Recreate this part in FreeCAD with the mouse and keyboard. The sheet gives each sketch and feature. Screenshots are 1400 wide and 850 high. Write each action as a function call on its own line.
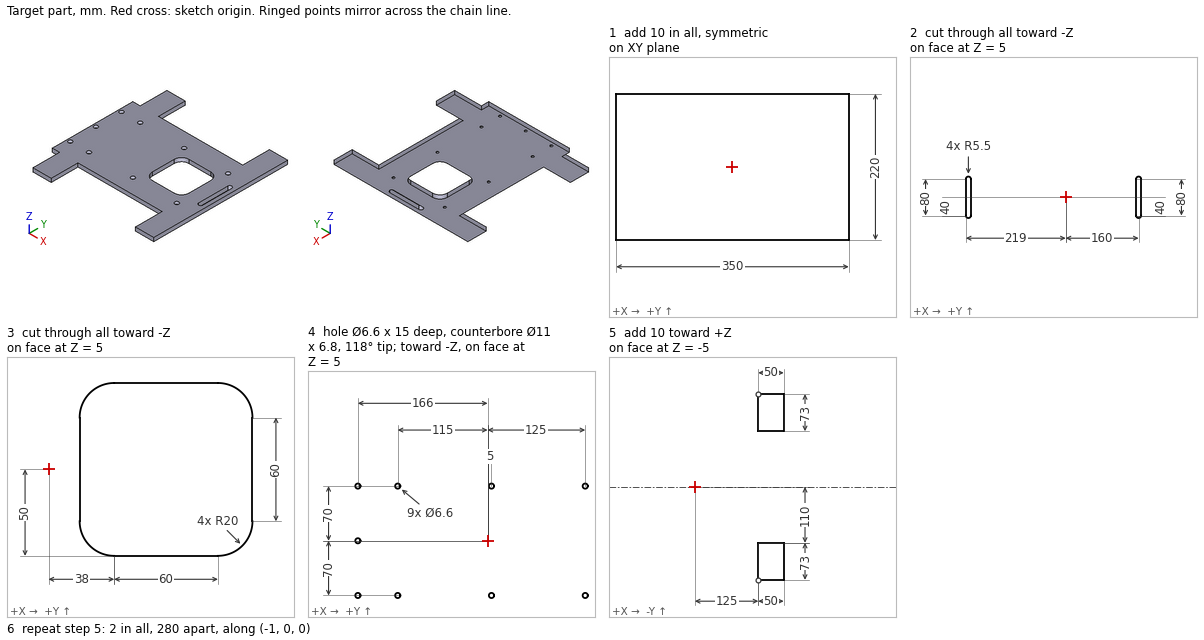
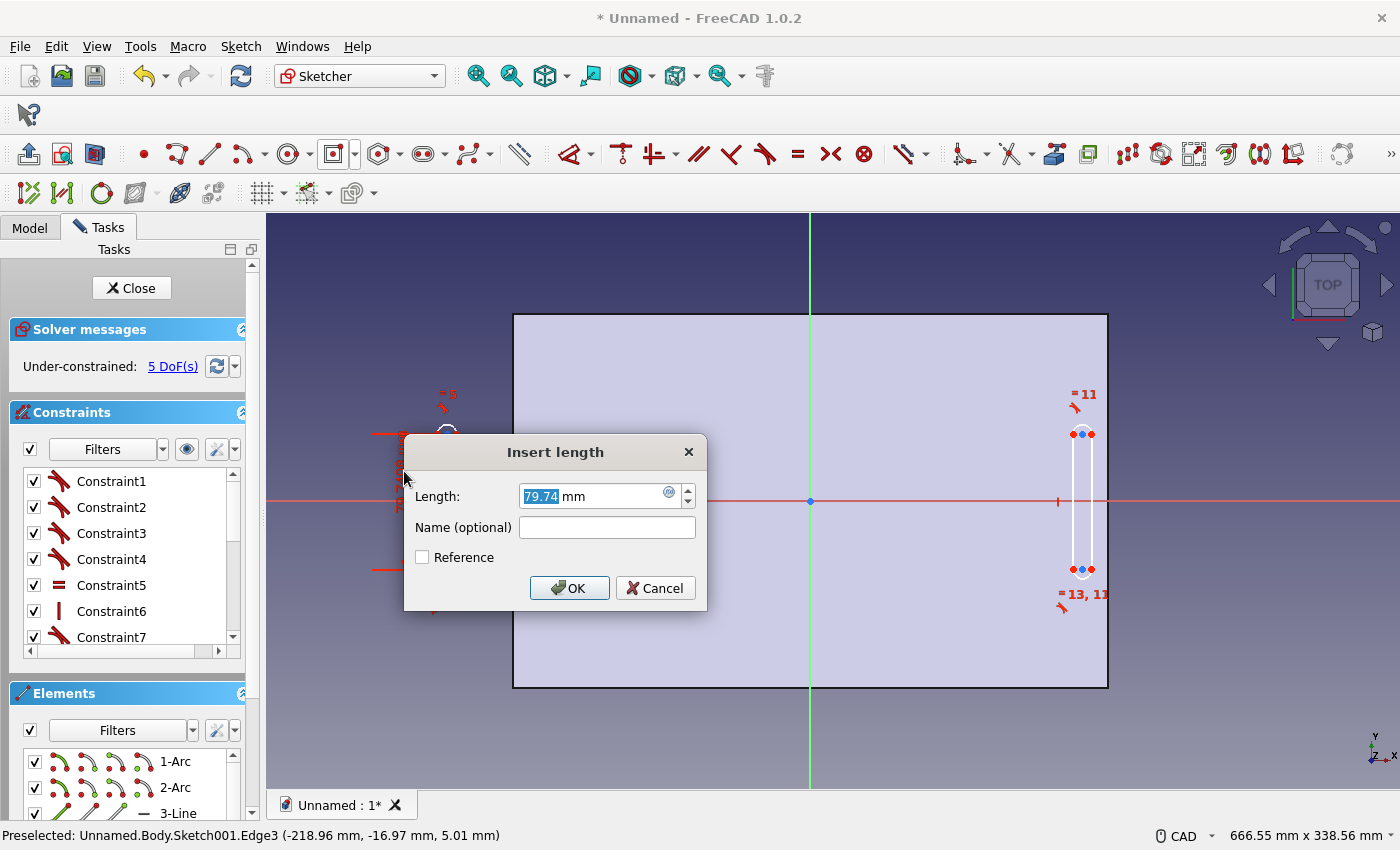
text(80)
key(Return)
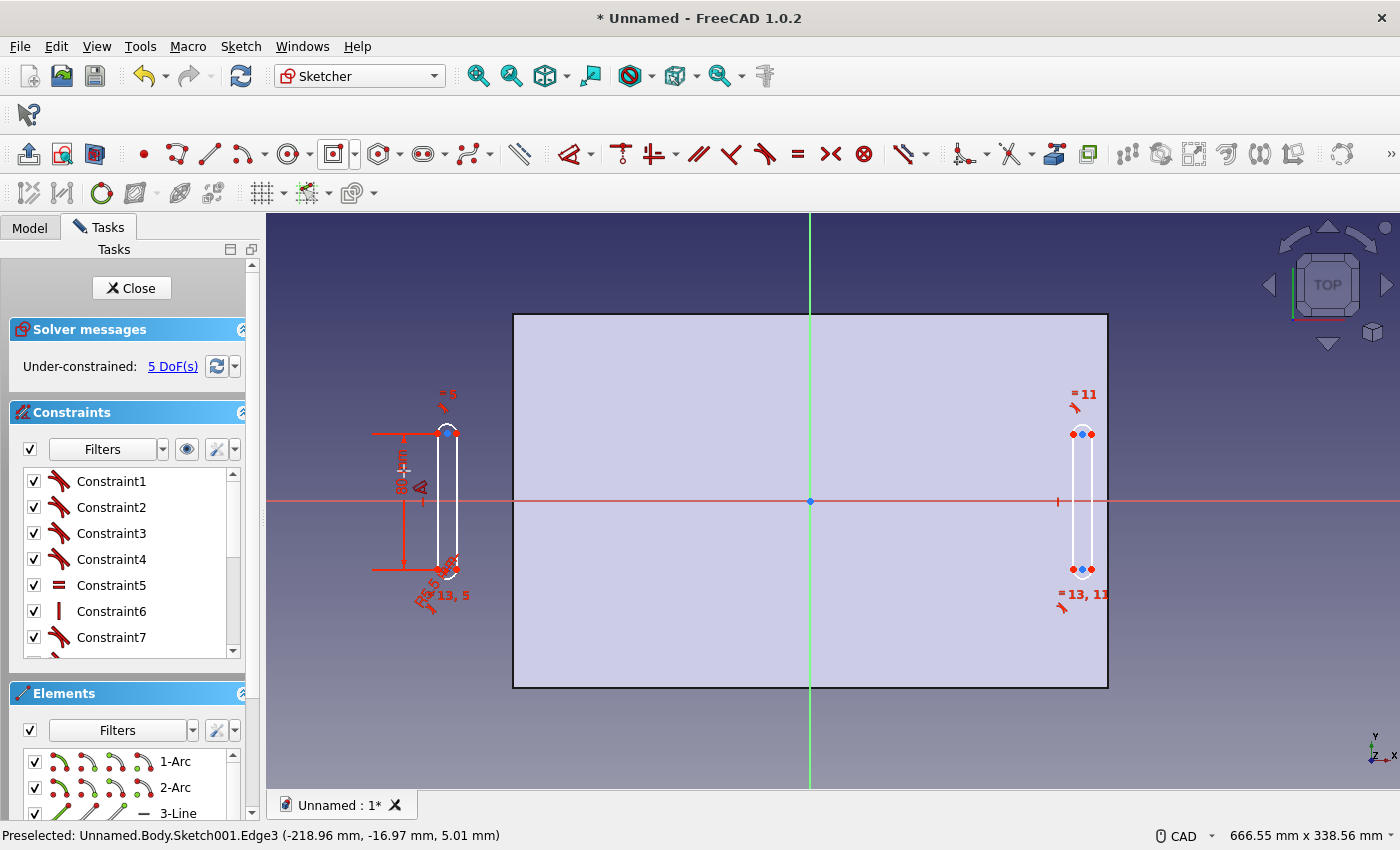
click(1073, 529)
click(1107, 471)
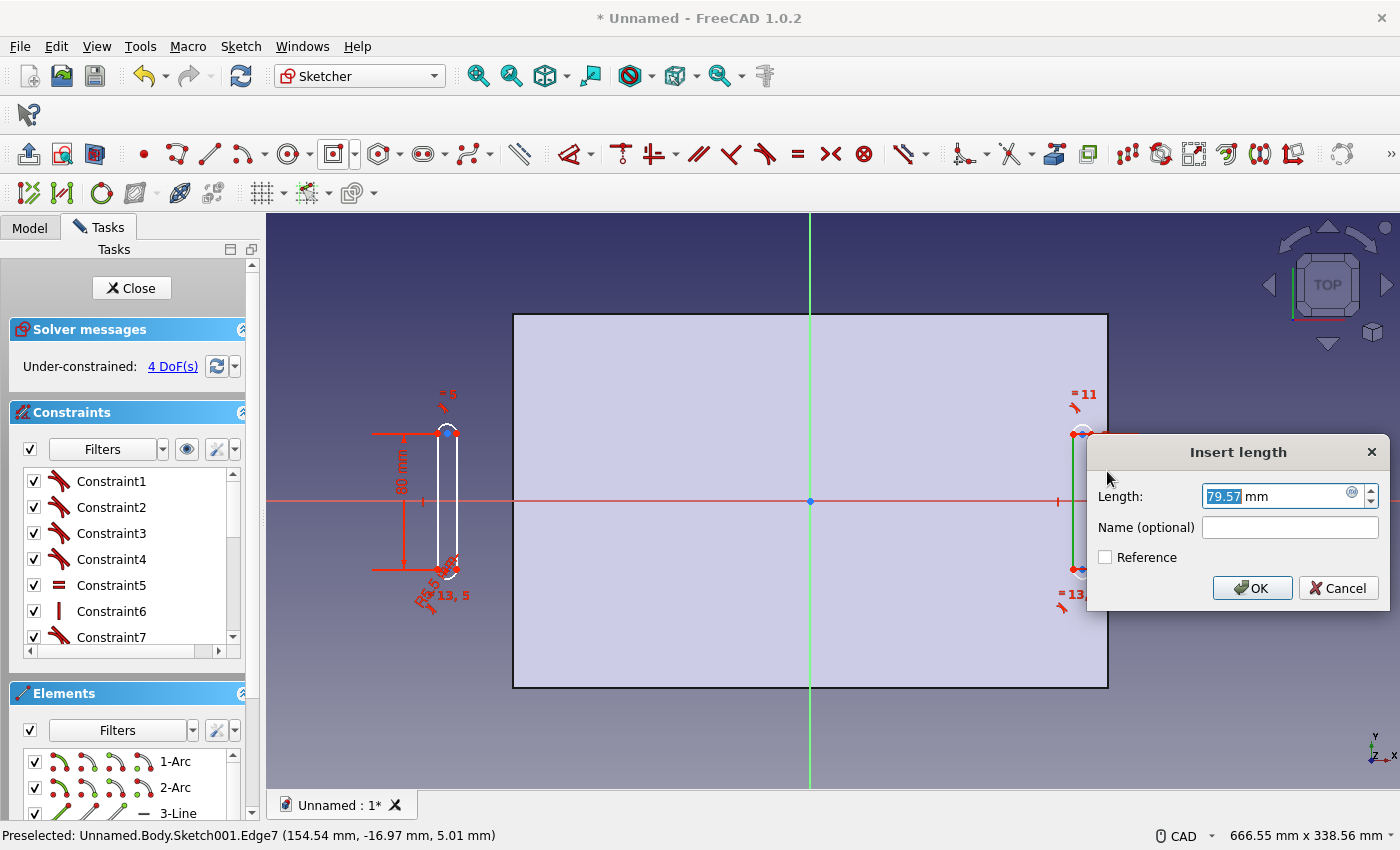
text(80)
key(Return)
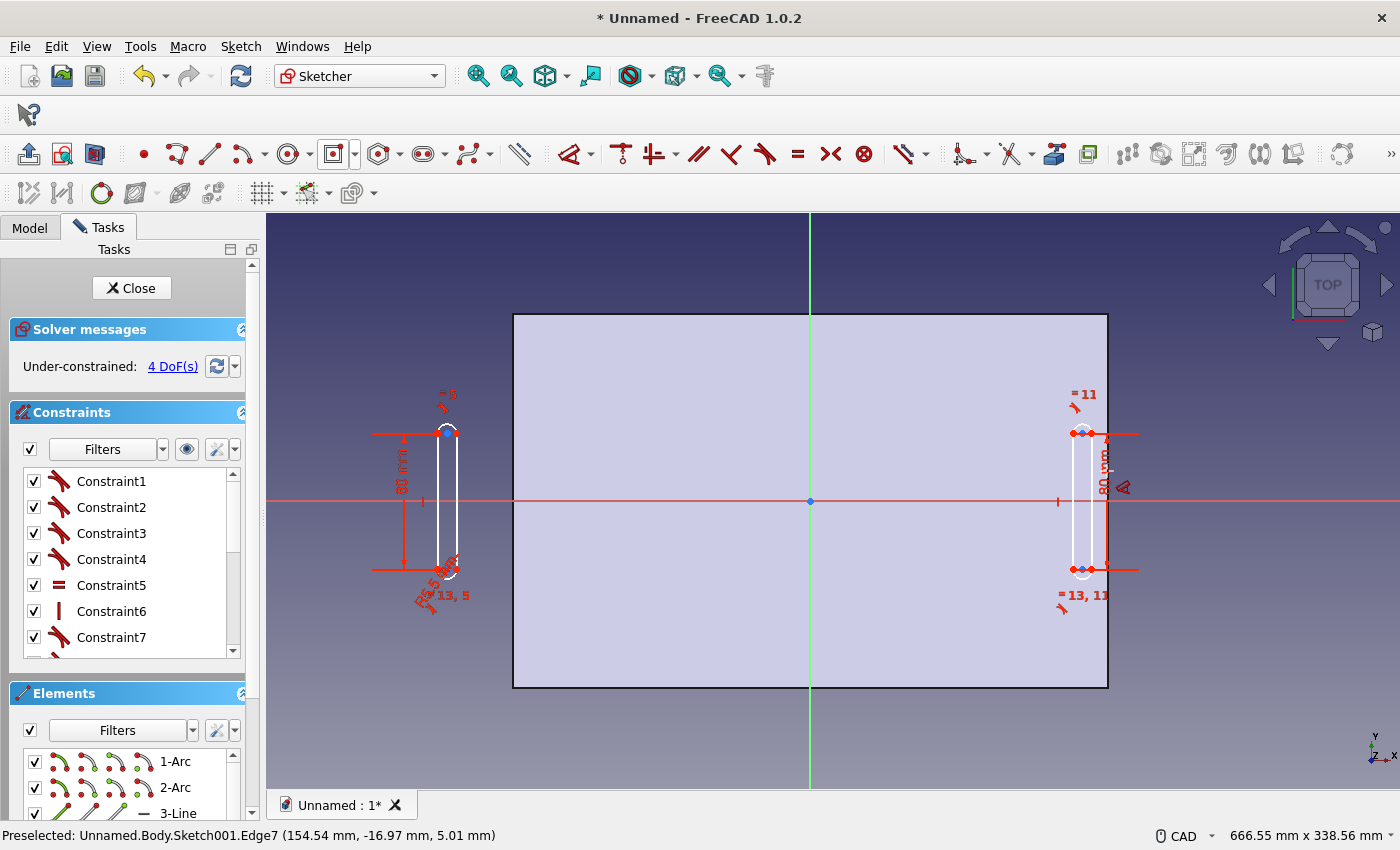
scroll(438, 570, up, 2)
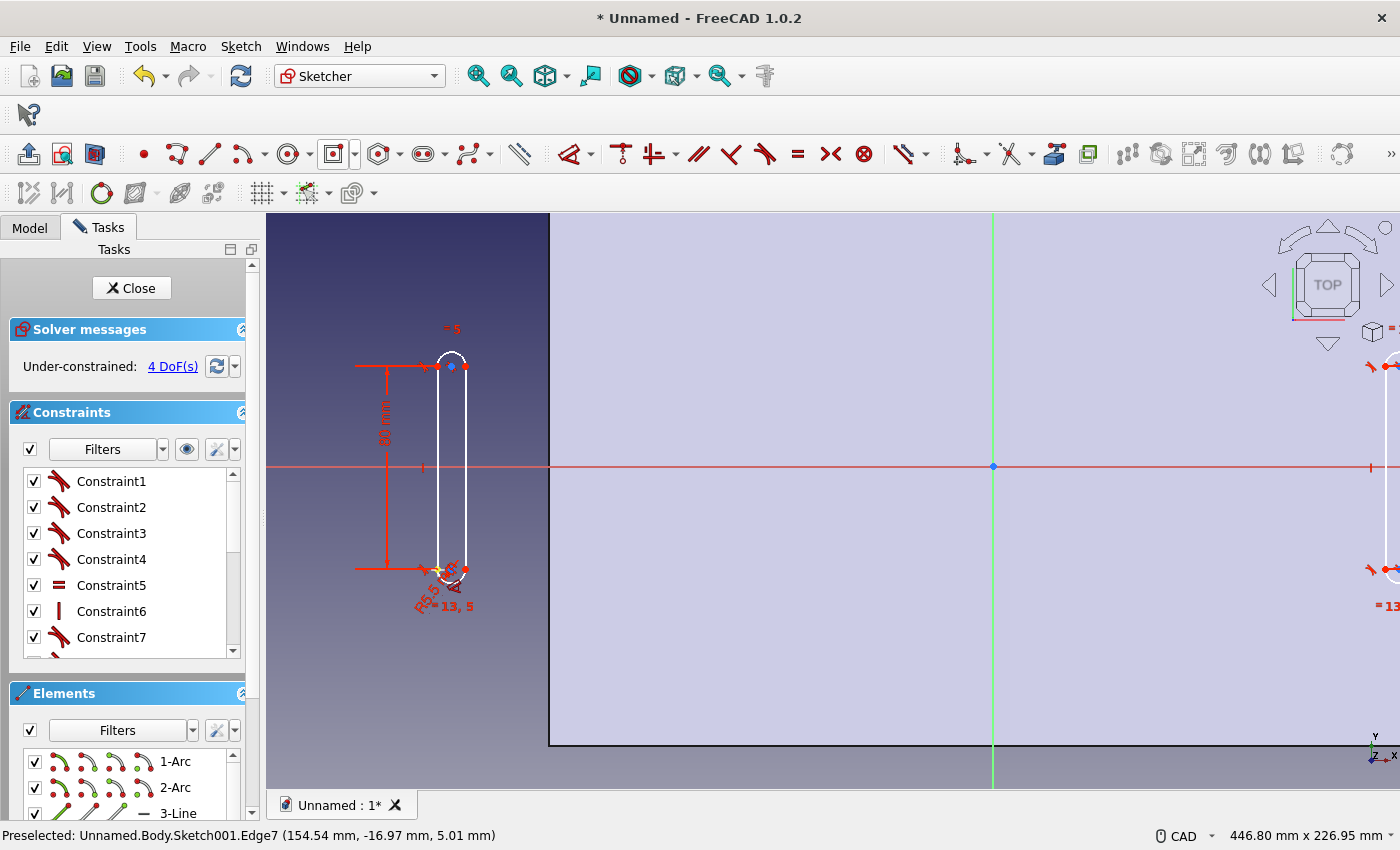
click(438, 569)
click(404, 518)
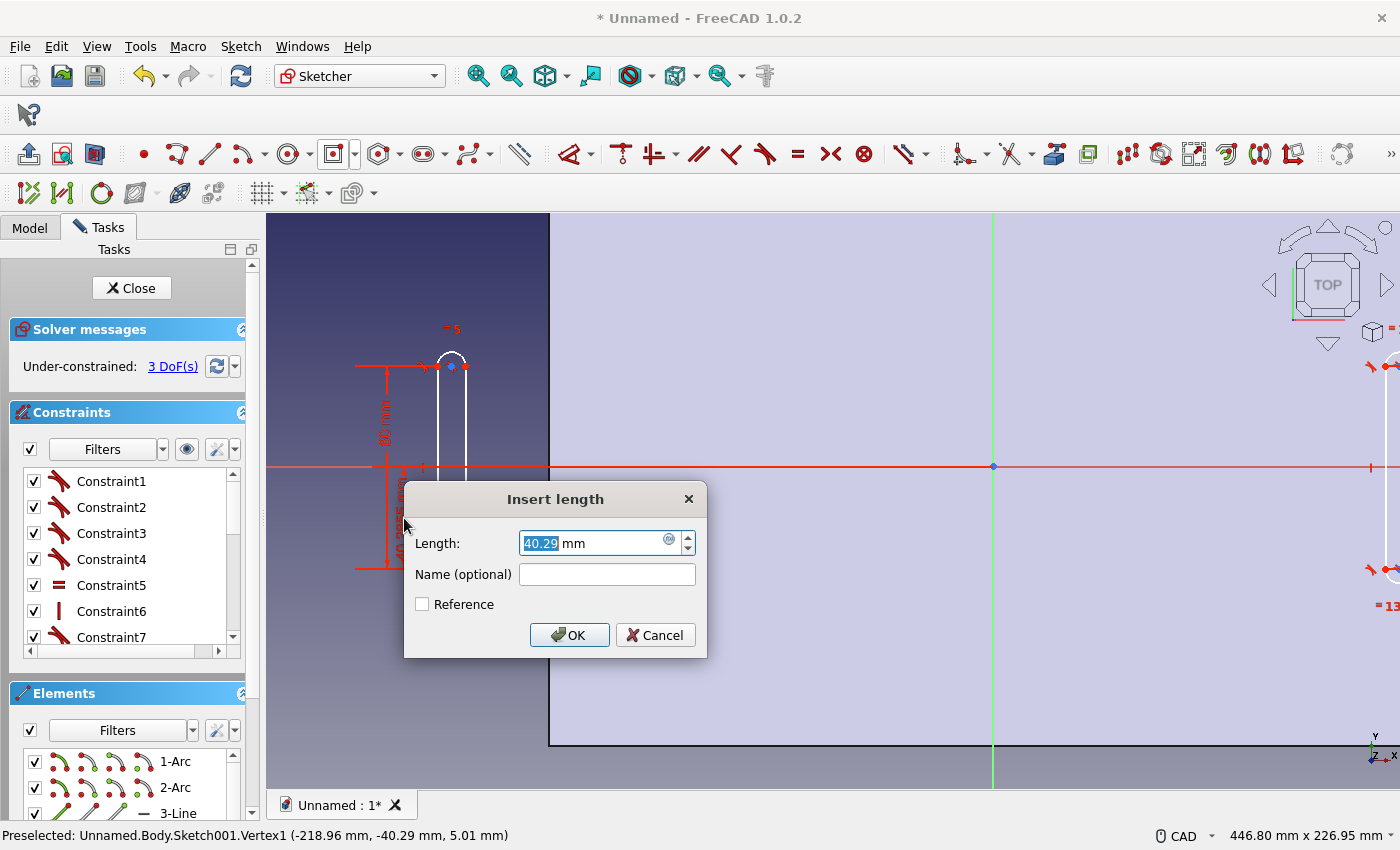
text(40)
key(Return)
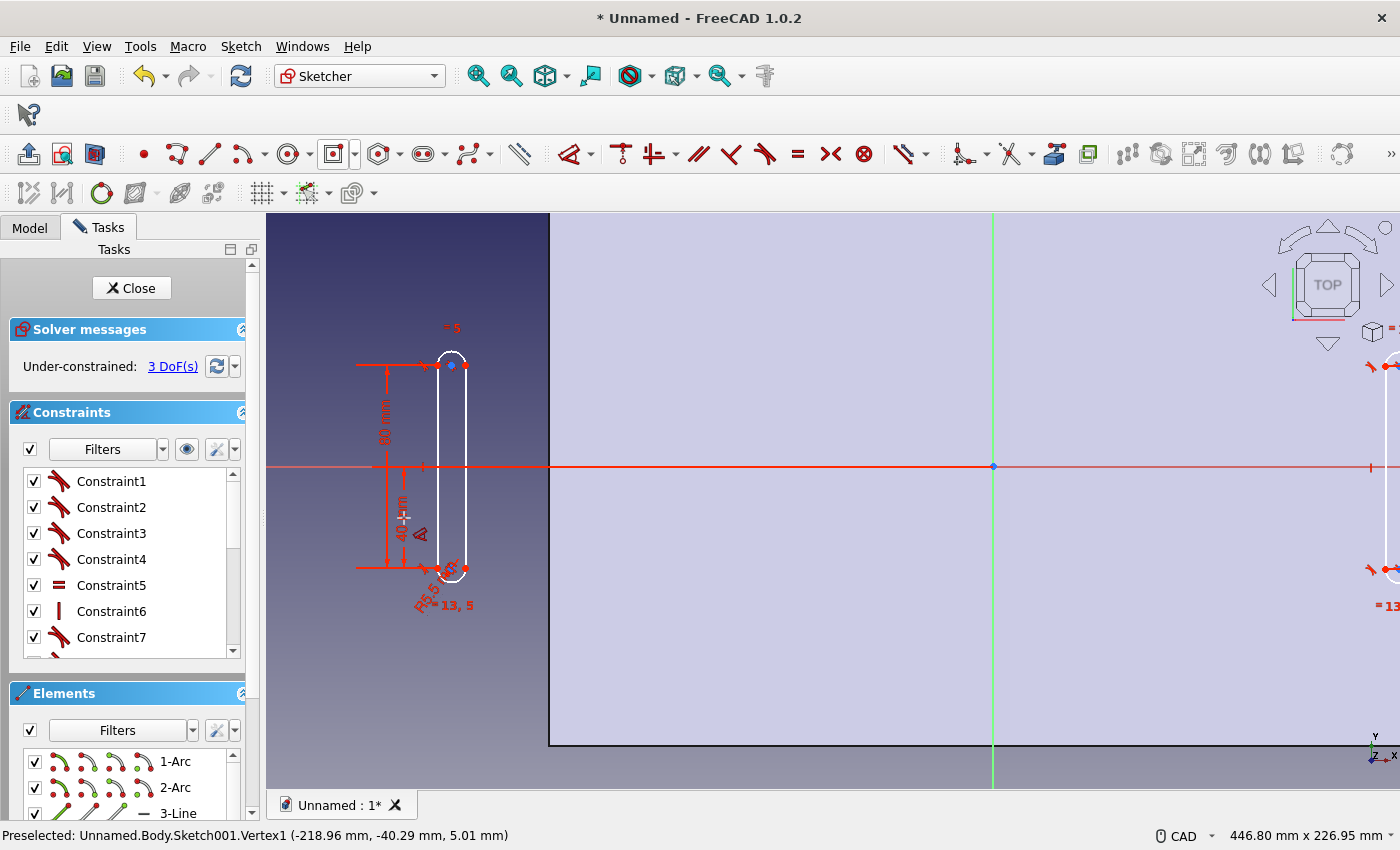
scroll(437, 570, down, 2)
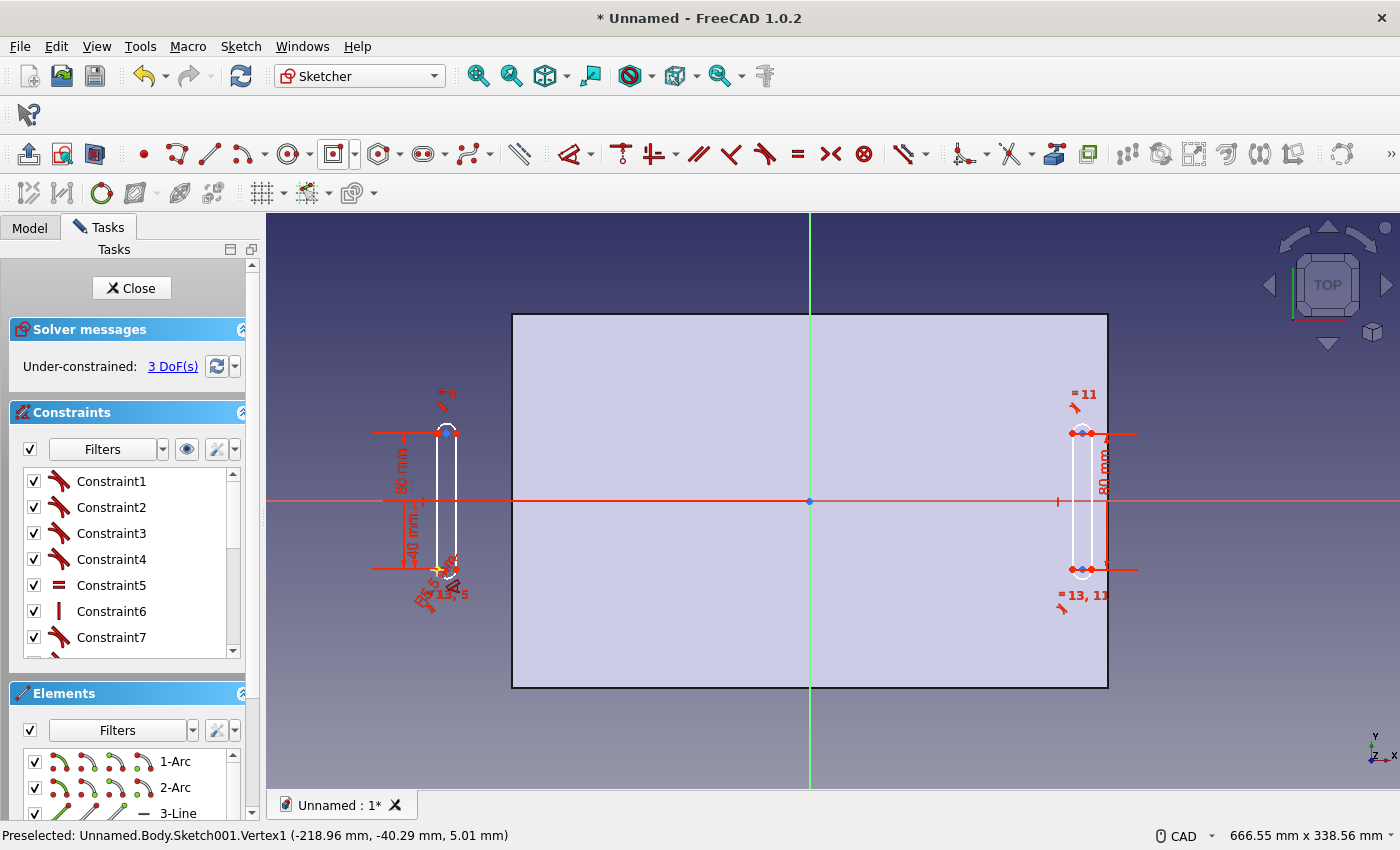
scroll(1073, 570, up, 2)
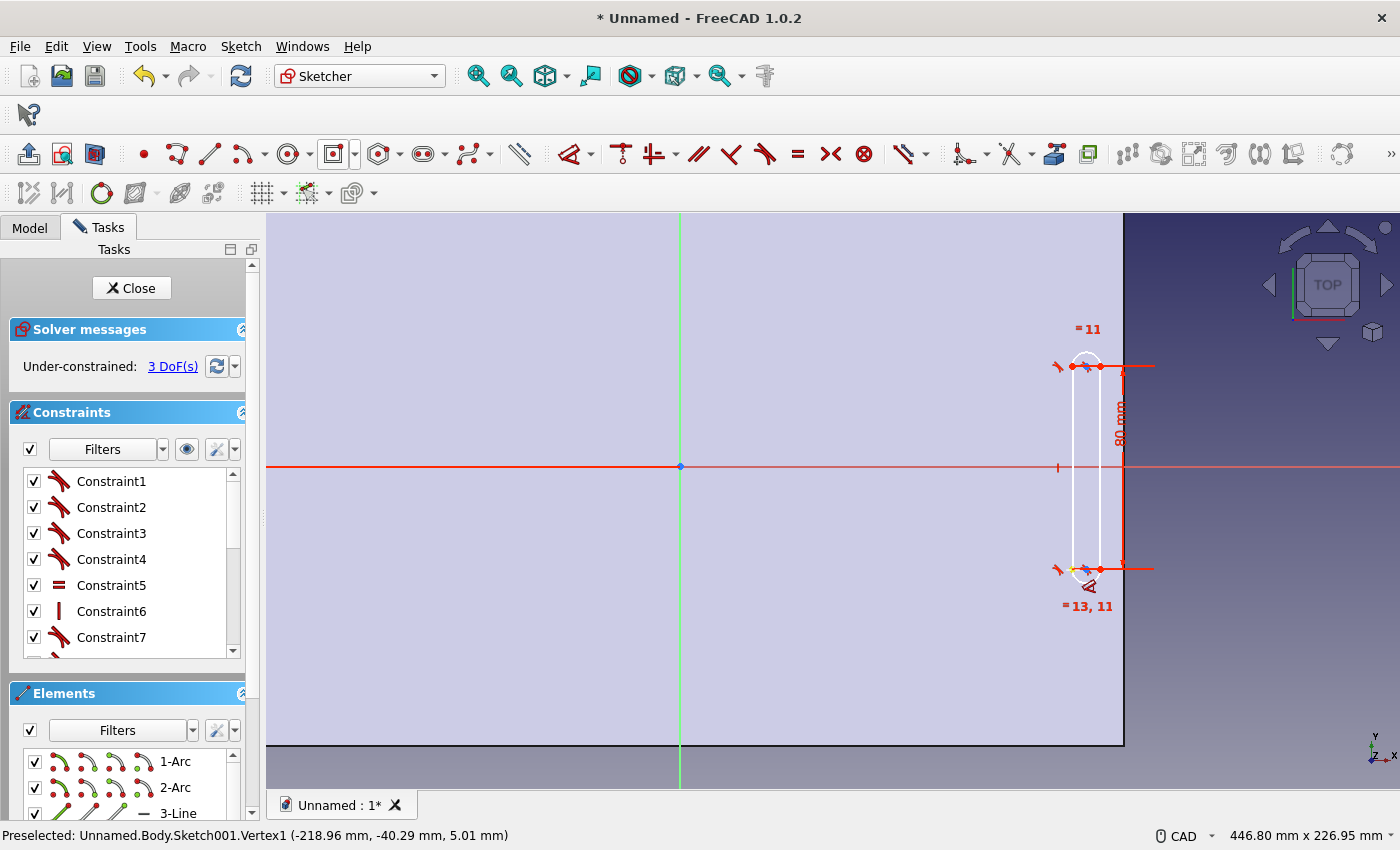
click(1073, 569)
click(646, 518)